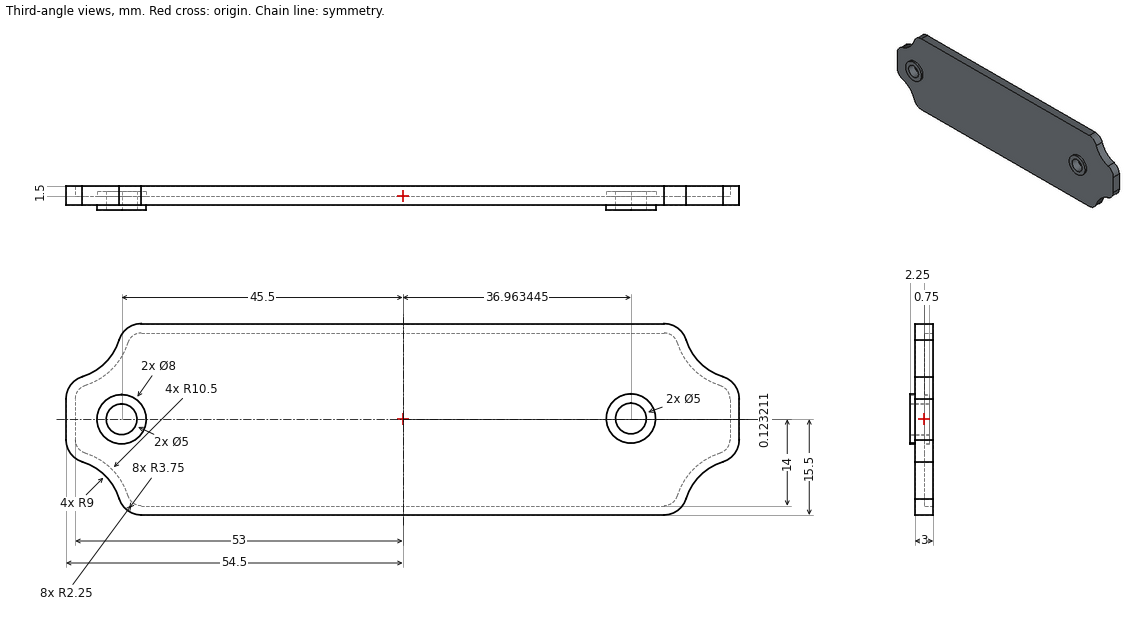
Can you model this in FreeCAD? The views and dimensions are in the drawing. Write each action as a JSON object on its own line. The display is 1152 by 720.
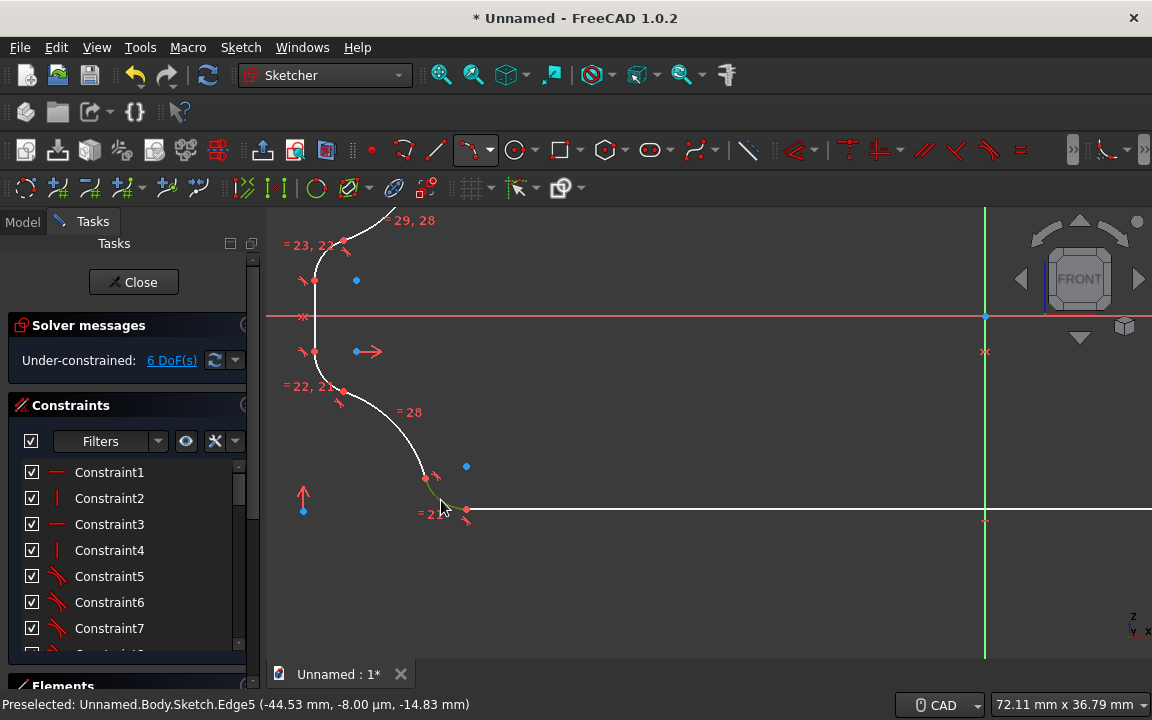
{"action": "key", "text": "k r"}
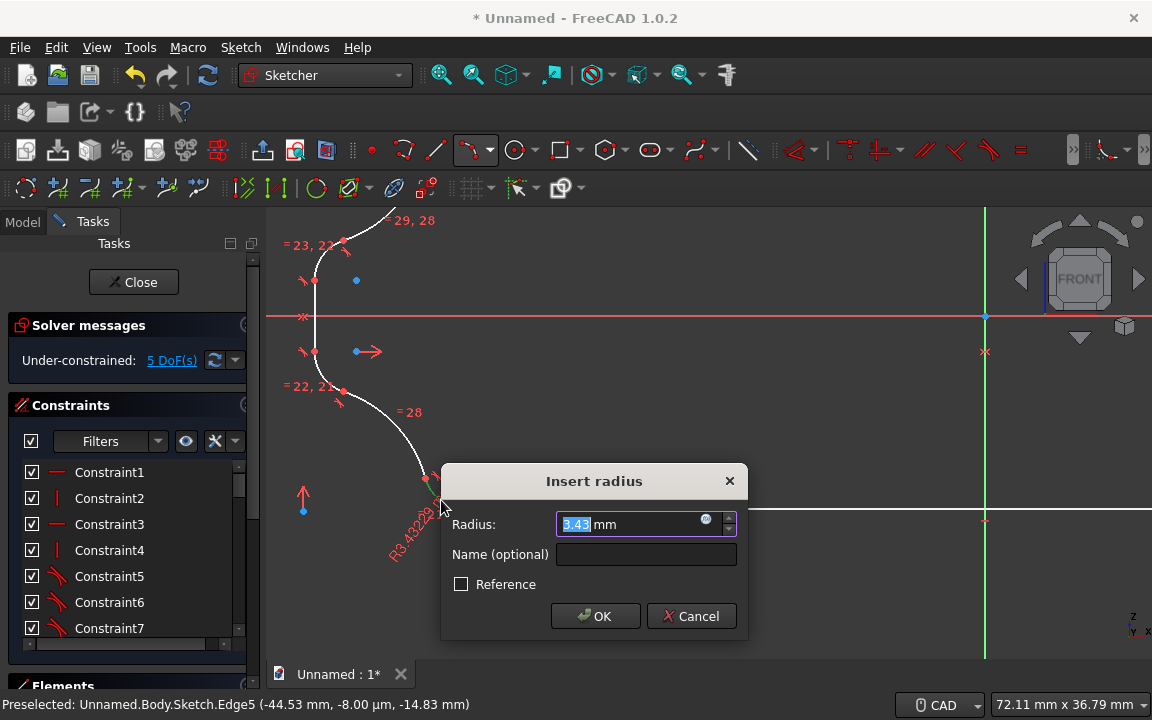
{"action": "type", "text": "3.75"}
{"action": "key", "text": "Return"}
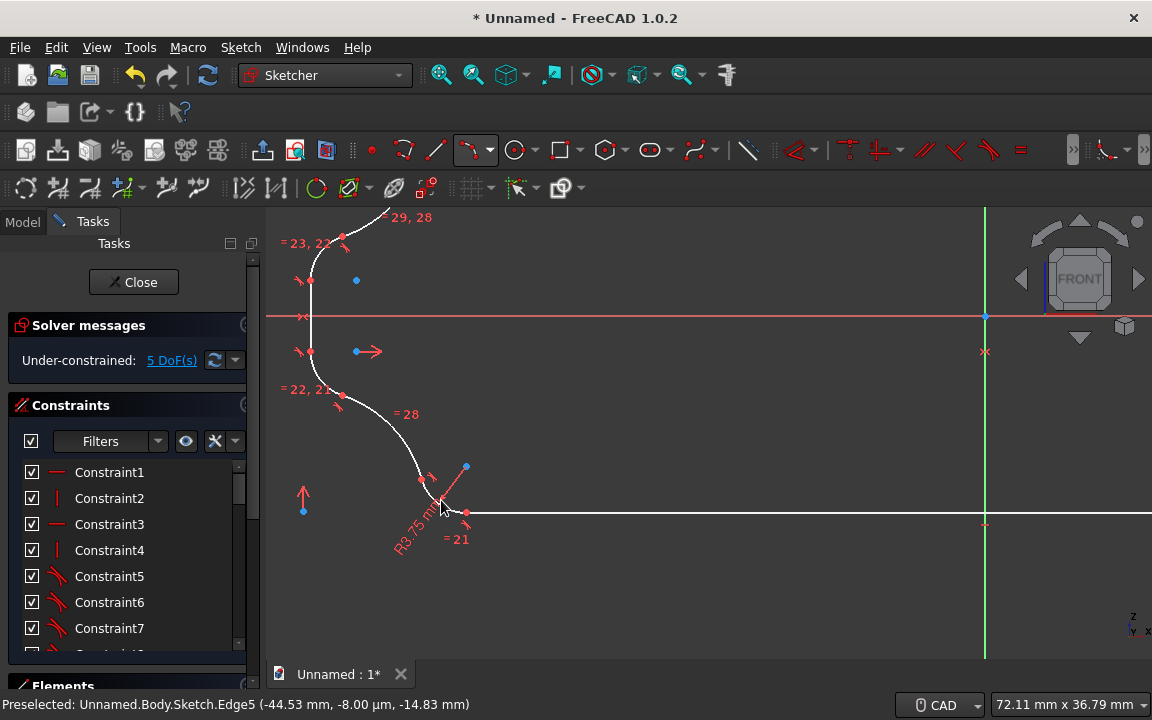
{"action": "left_click", "coordinate": [407, 446]}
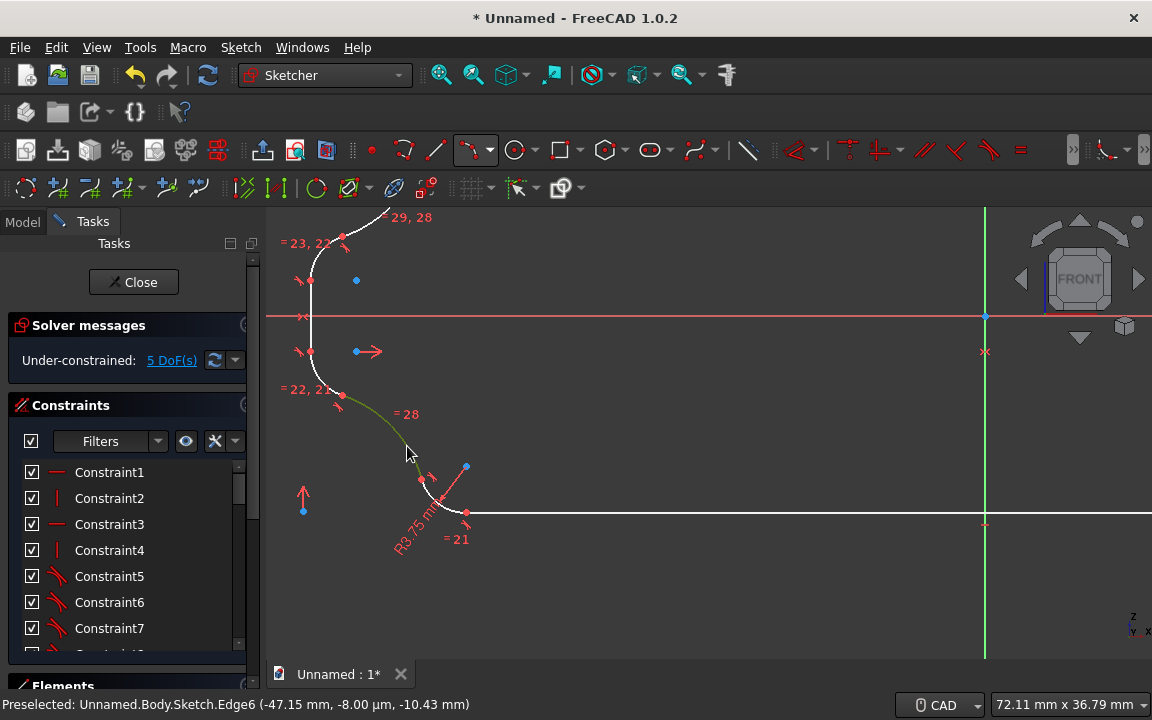
{"action": "key", "text": "k r"}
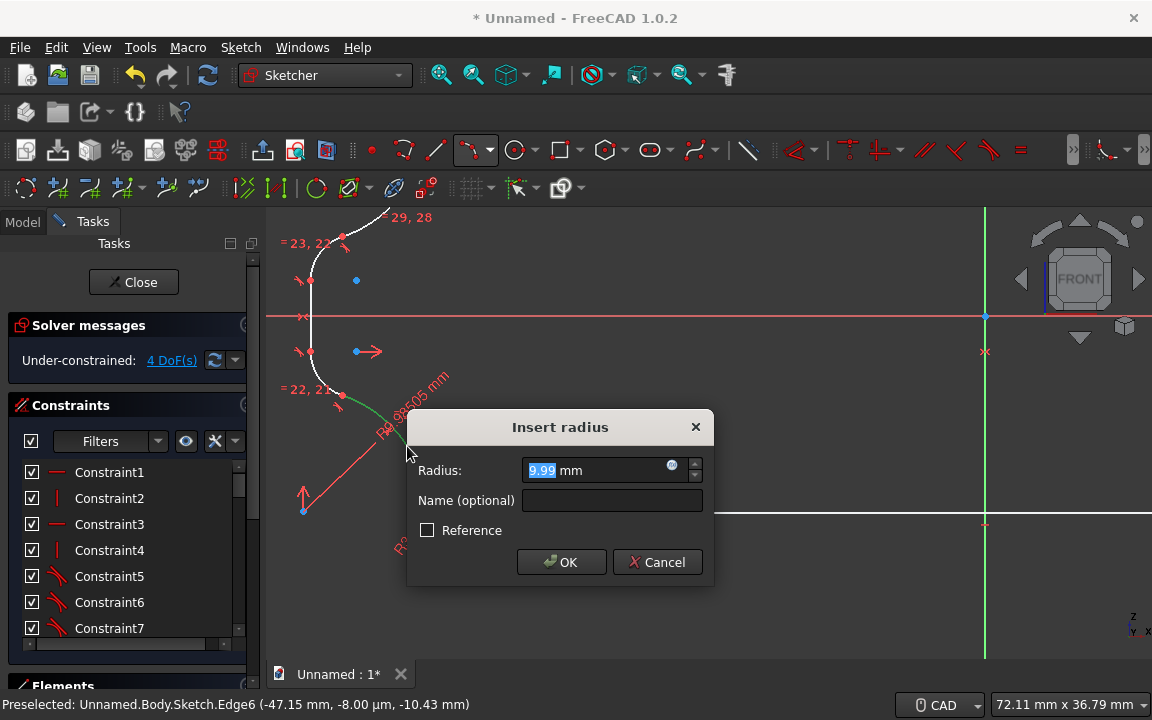
{"action": "type", "text": "9"}
{"action": "key", "text": "Return"}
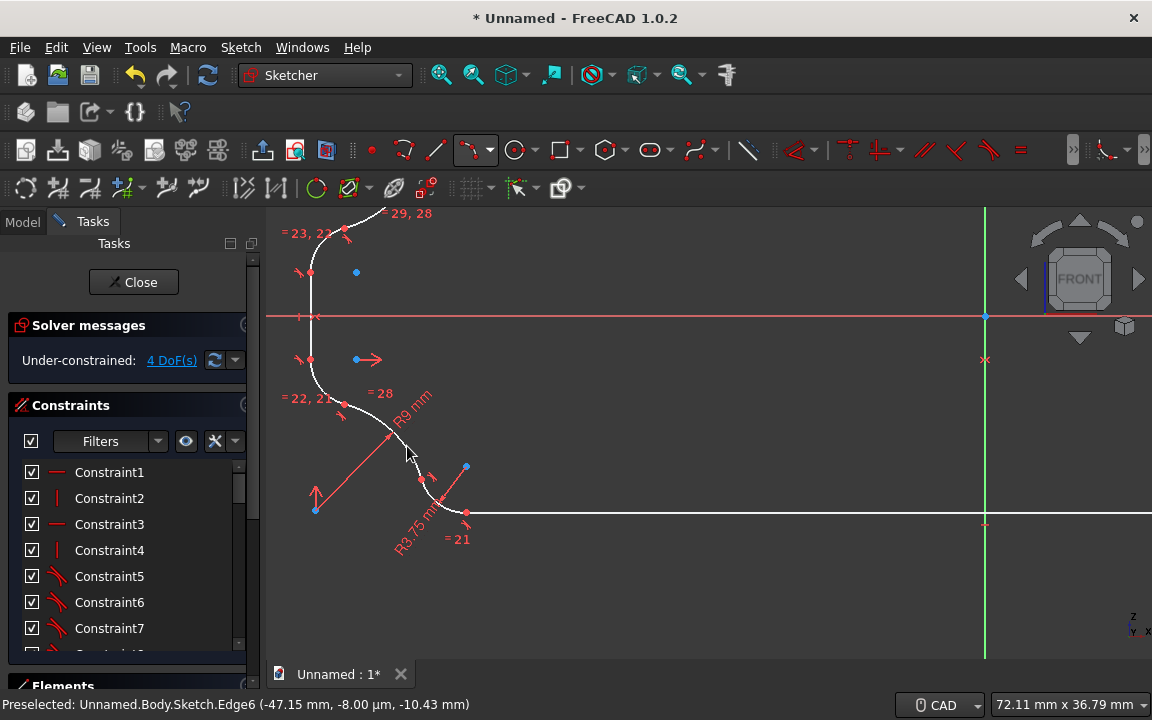
{"action": "scroll", "coordinate": [440, 501], "scroll_direction": "down", "scroll_amount": 5}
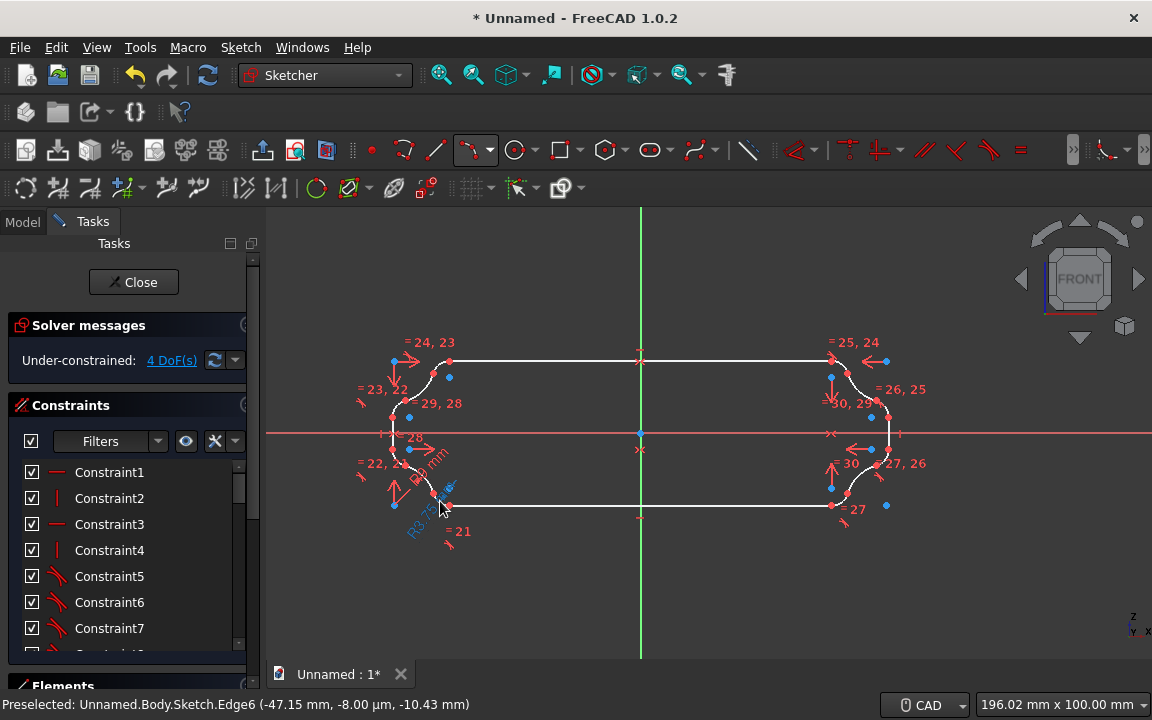
{"action": "left_click", "coordinate": [832, 506]}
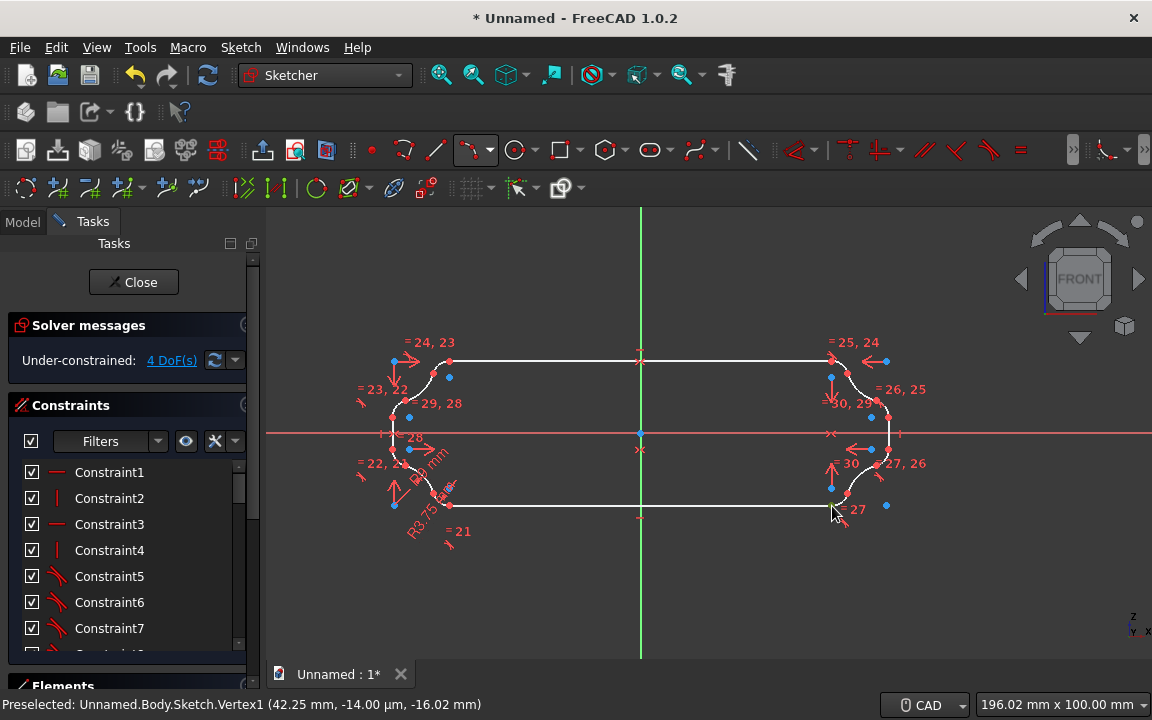
{"action": "left_click", "coordinate": [816, 150]}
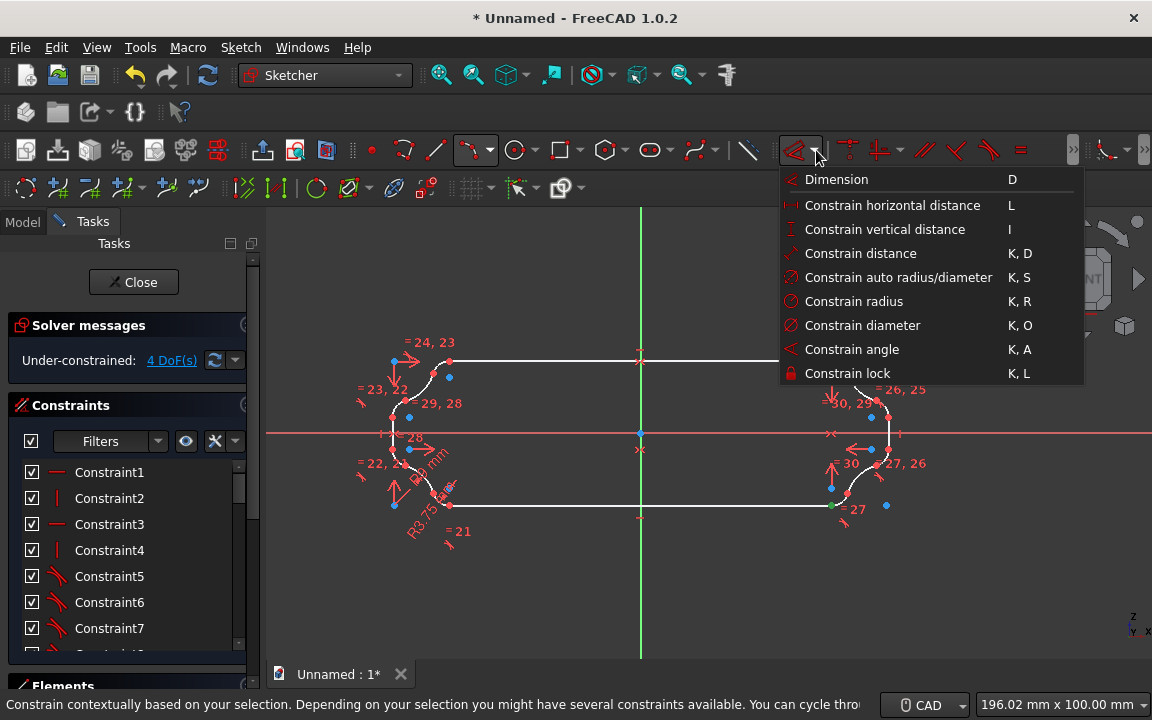
{"action": "left_click", "coordinate": [932, 229]}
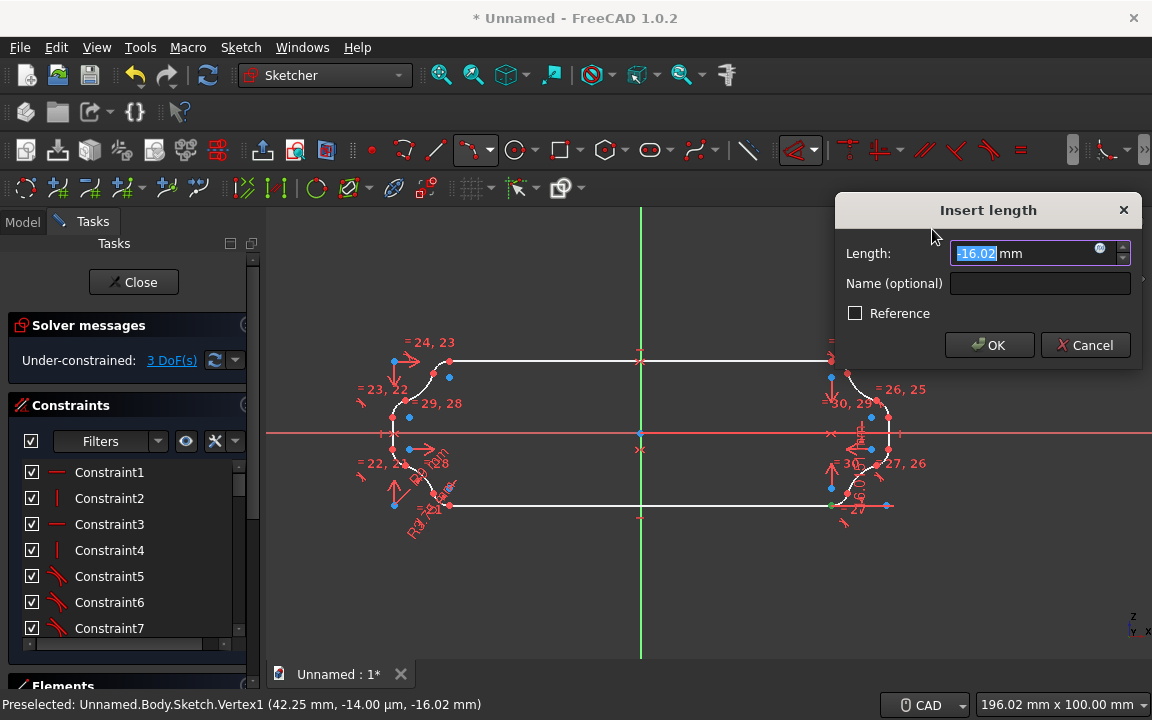
{"action": "type", "text": "-15.5"}
{"action": "key", "text": "Return"}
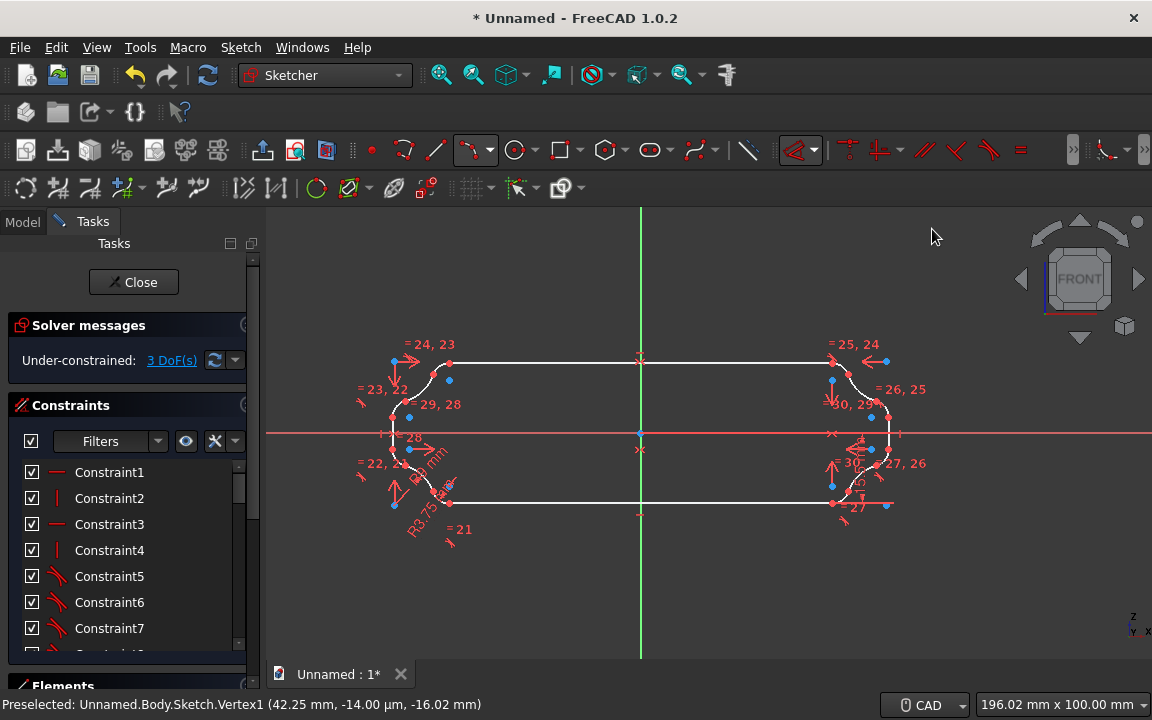
{"action": "left_click", "coordinate": [393, 449]}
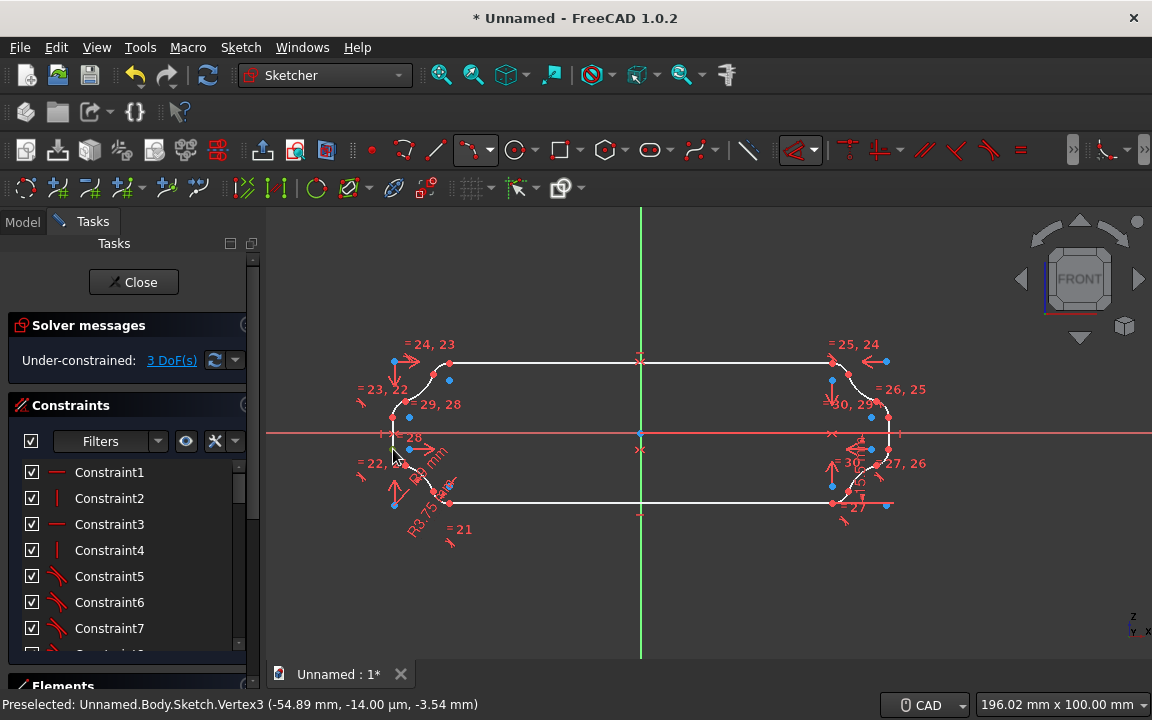
{"action": "key", "text": "l"}